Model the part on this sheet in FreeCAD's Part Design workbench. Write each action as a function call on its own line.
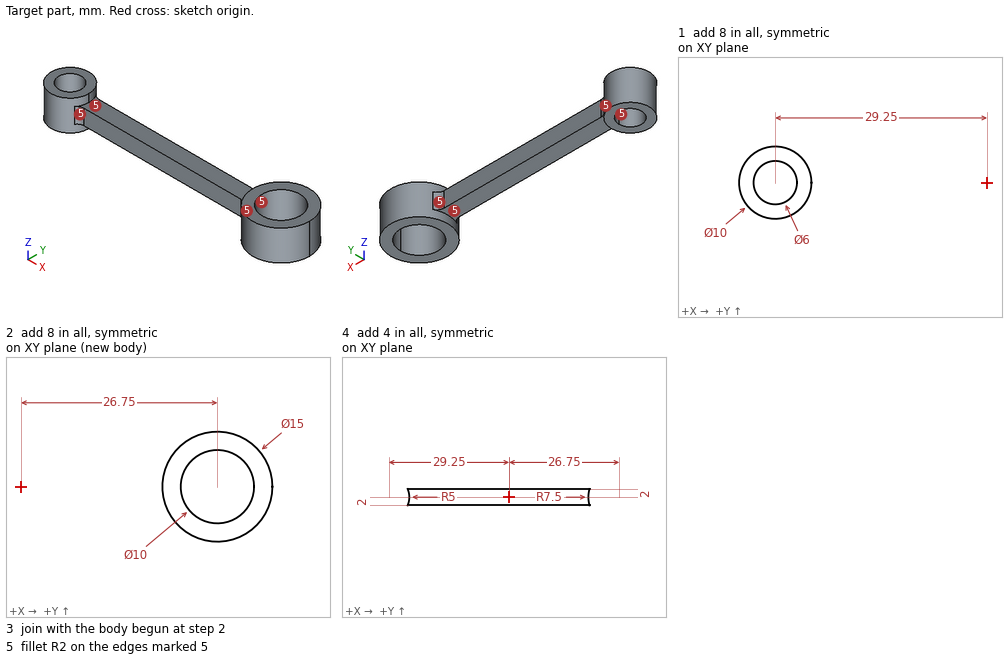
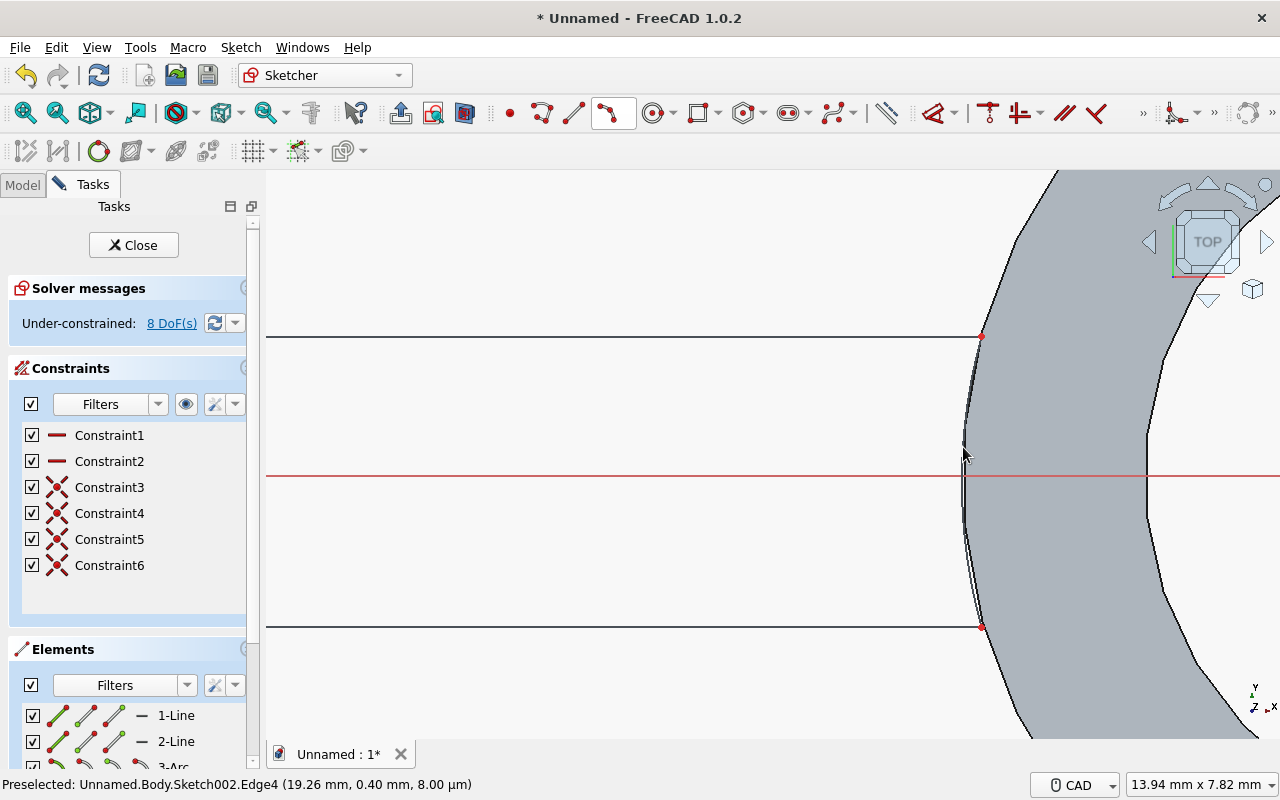
scroll(968, 450, down, 9)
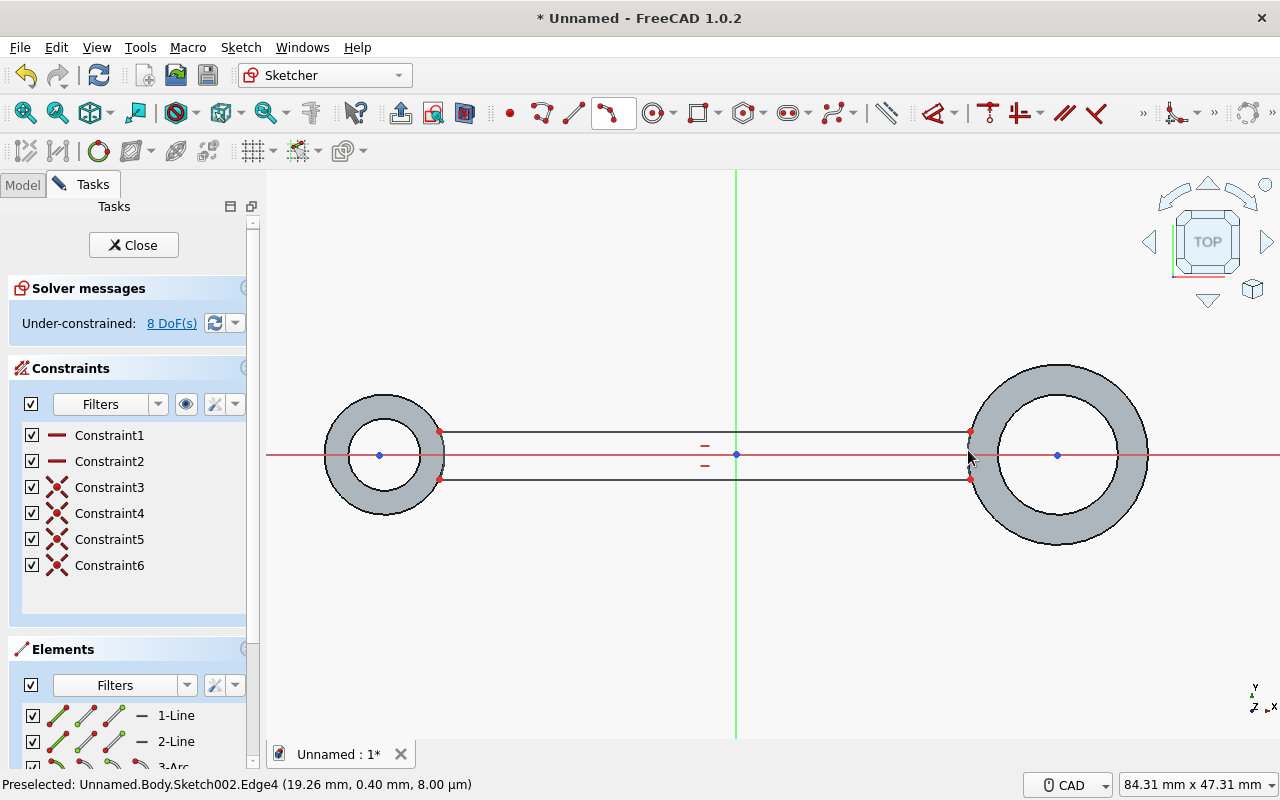
click(379, 456)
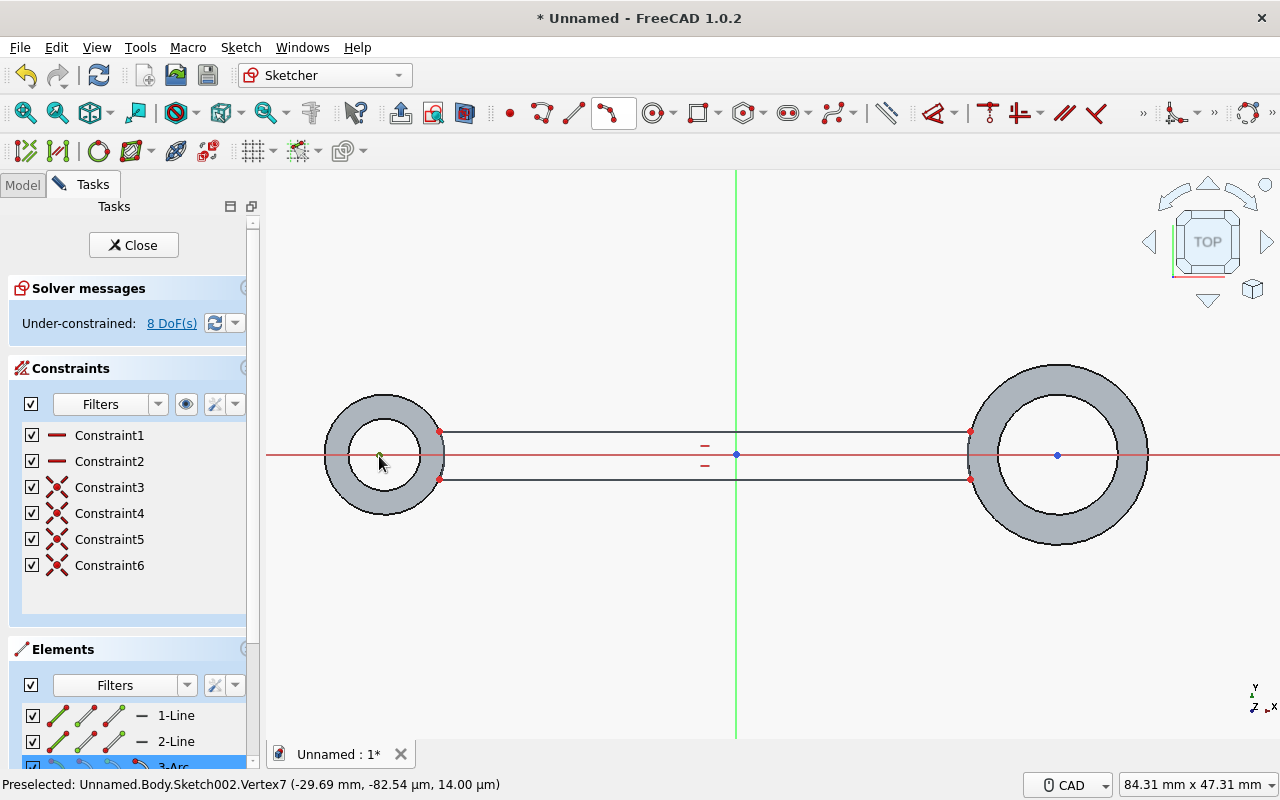
click(353, 455)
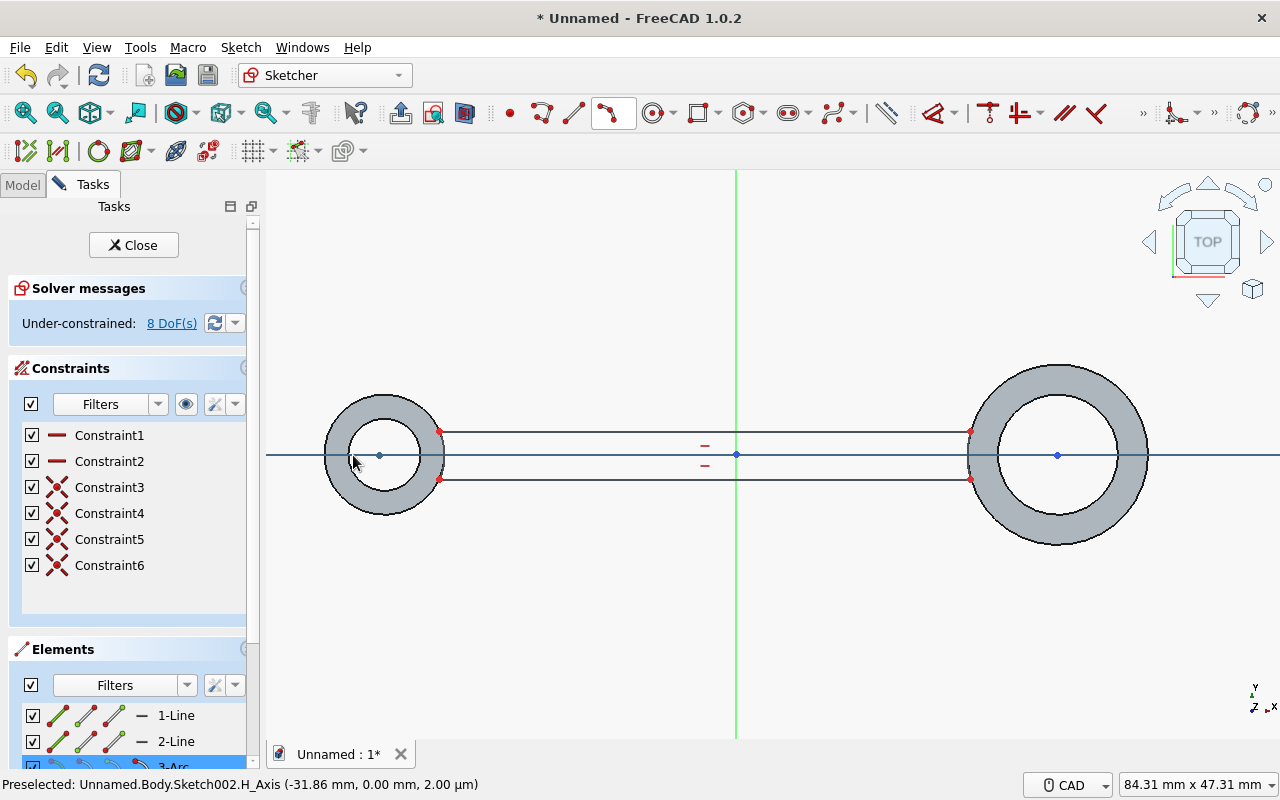
click(988, 114)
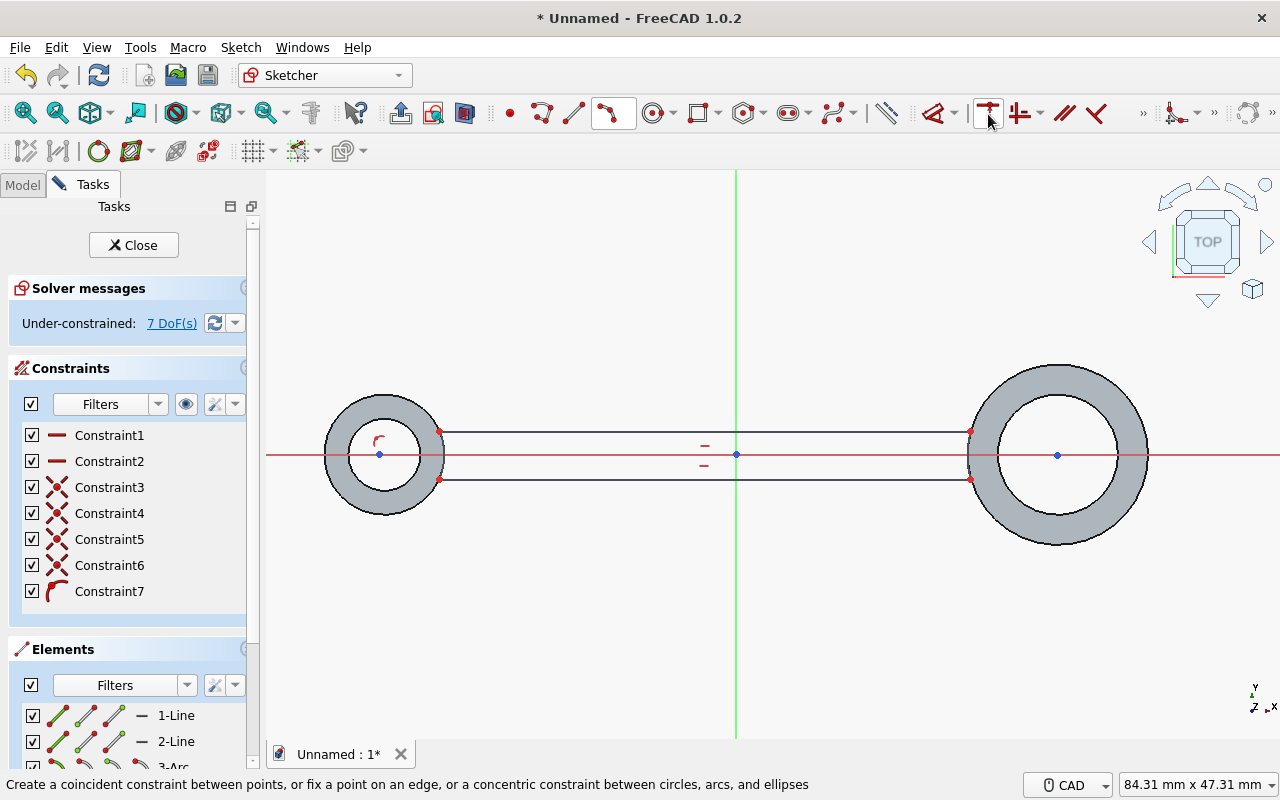
click(1058, 456)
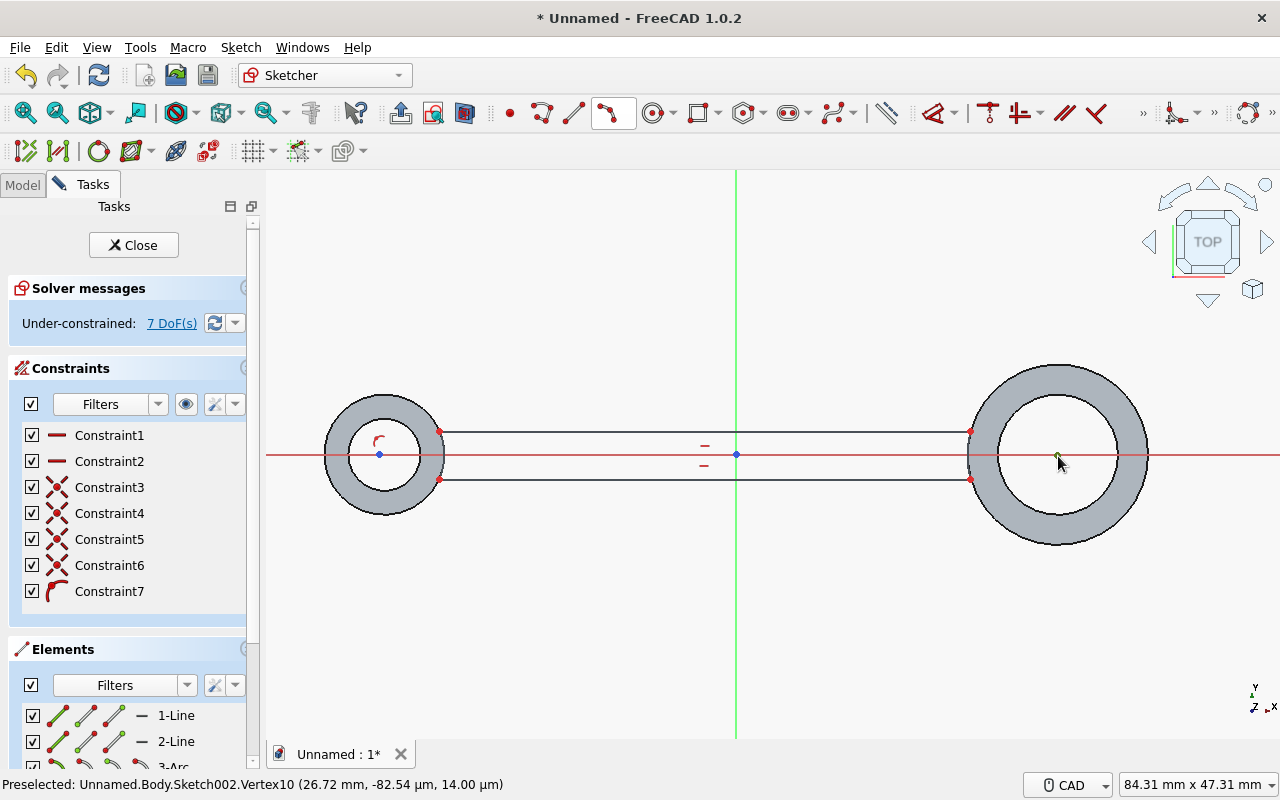
click(353, 455)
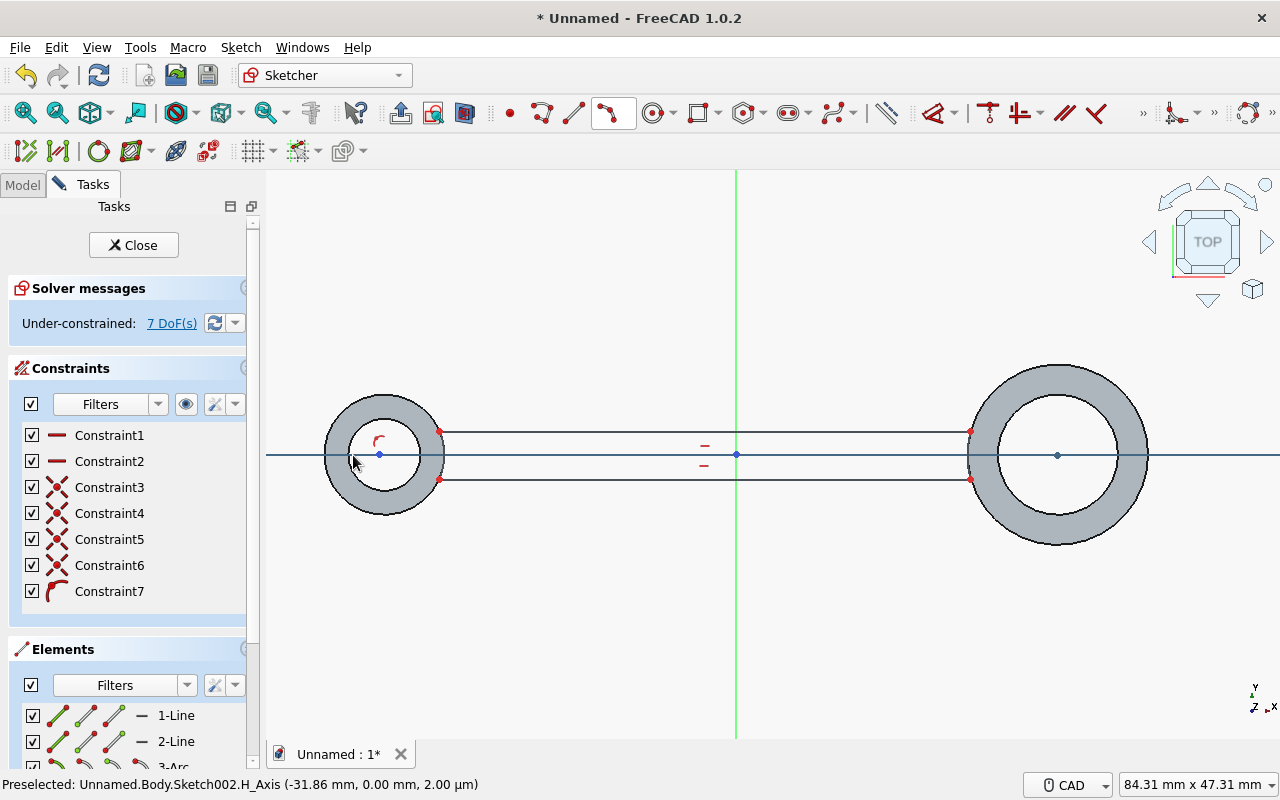
click(988, 114)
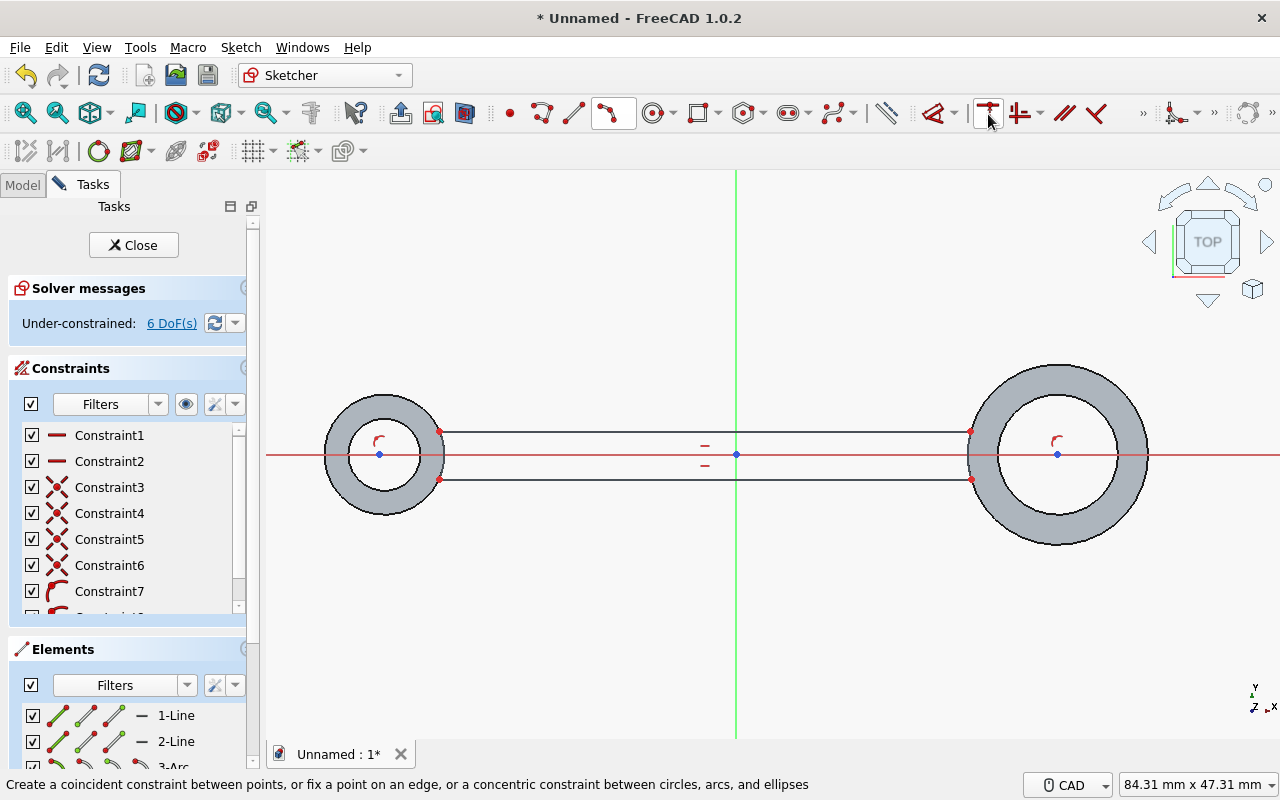
click(934, 114)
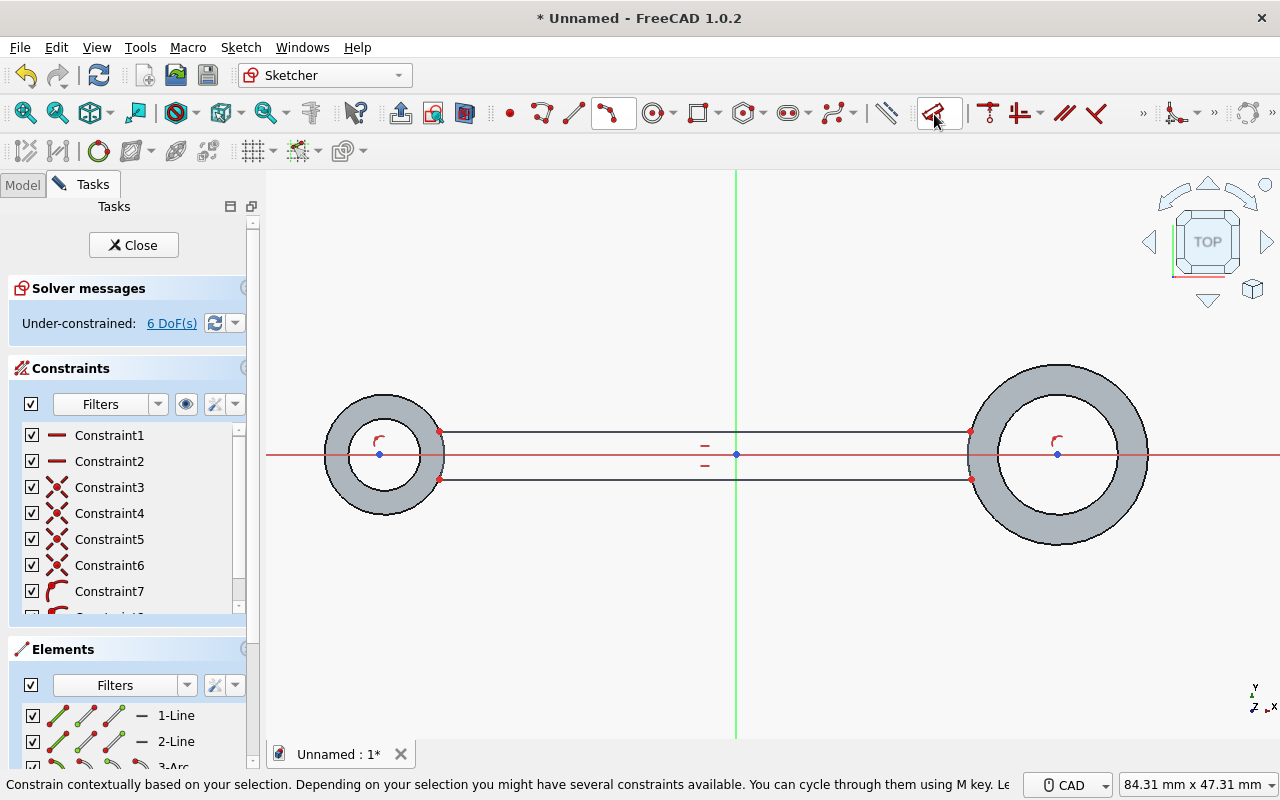
scroll(443, 466, up, 2)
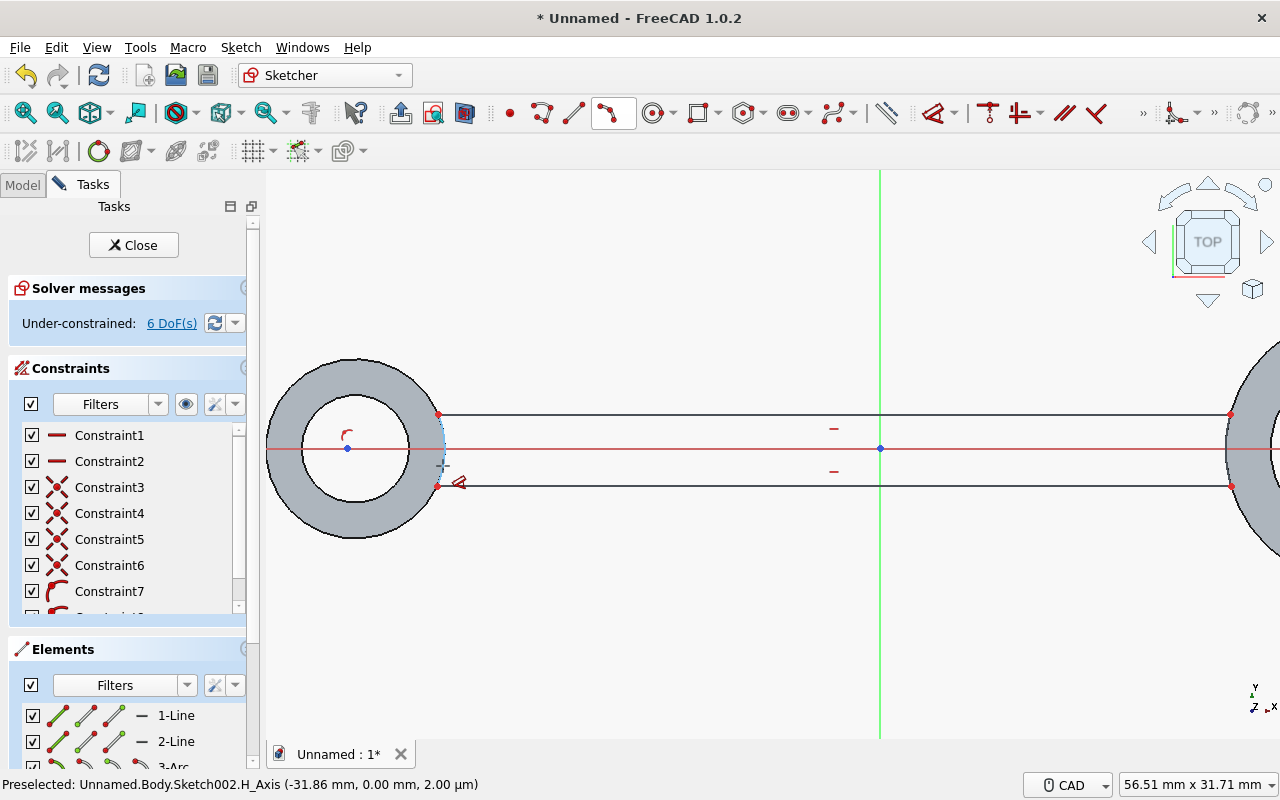
click(443, 465)
click(475, 470)